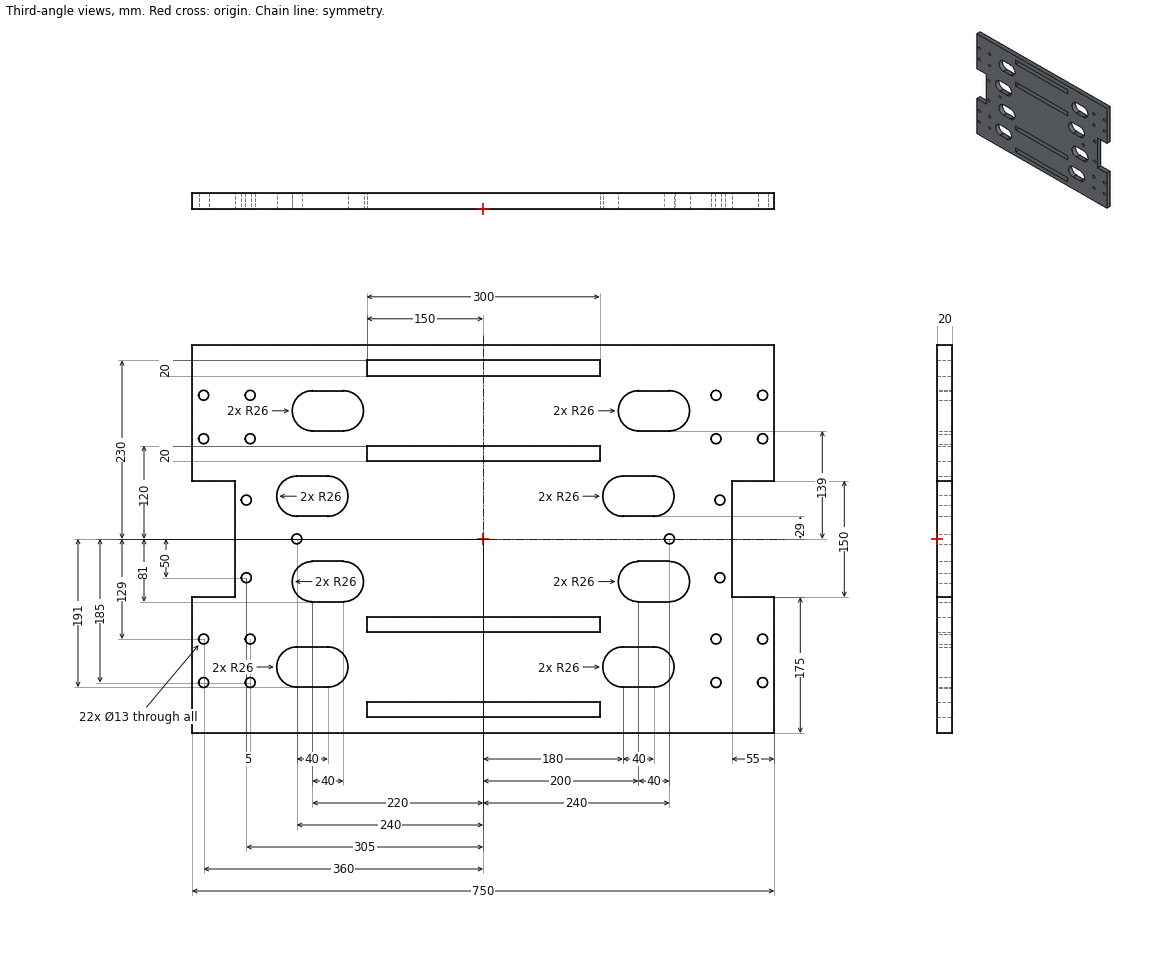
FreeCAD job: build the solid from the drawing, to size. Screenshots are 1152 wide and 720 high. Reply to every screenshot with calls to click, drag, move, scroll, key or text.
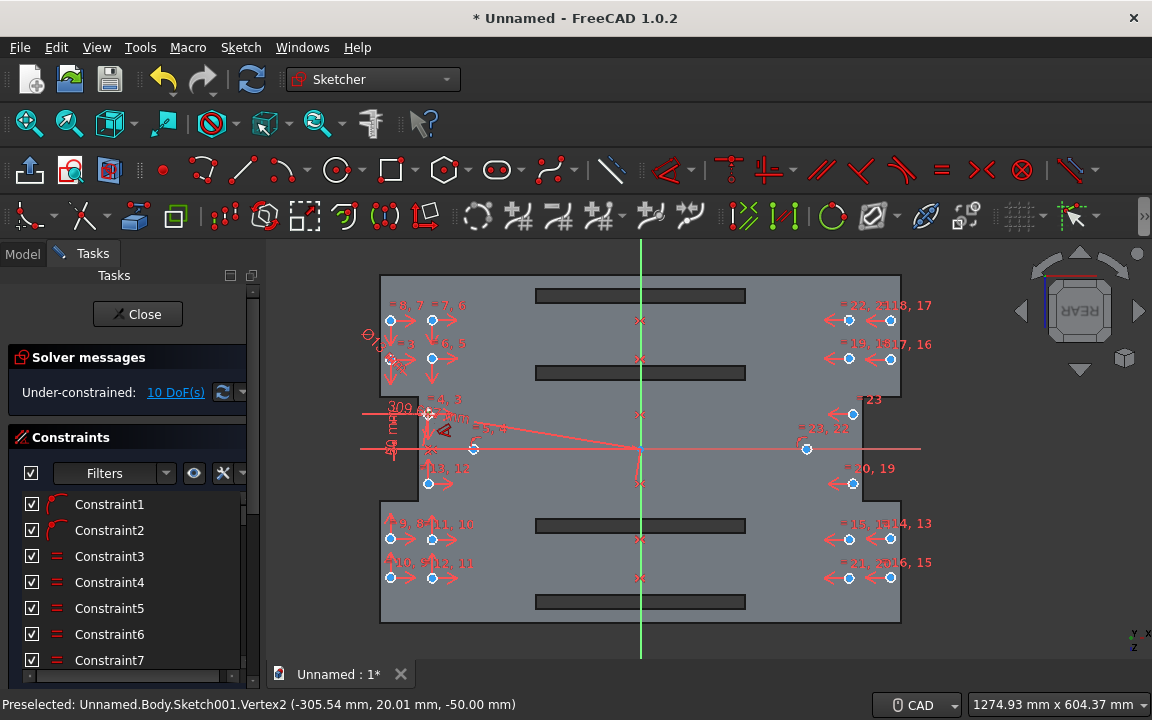
scroll(432, 359, up, 13)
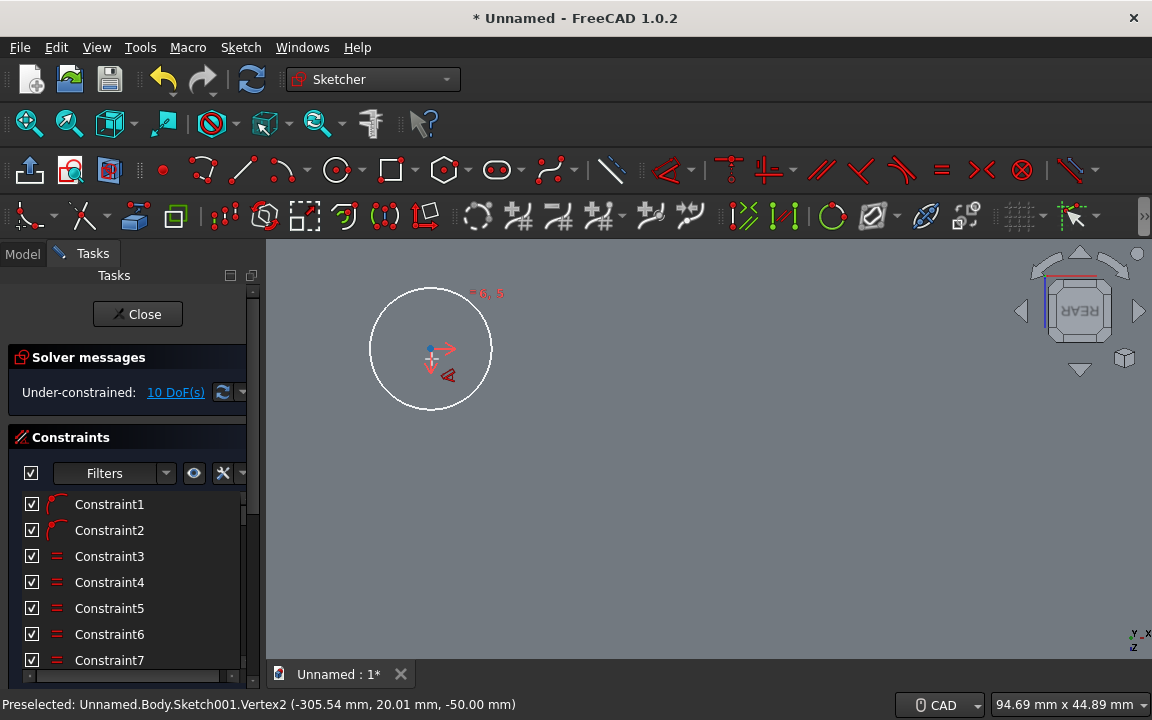
click(431, 349)
click(406, 315)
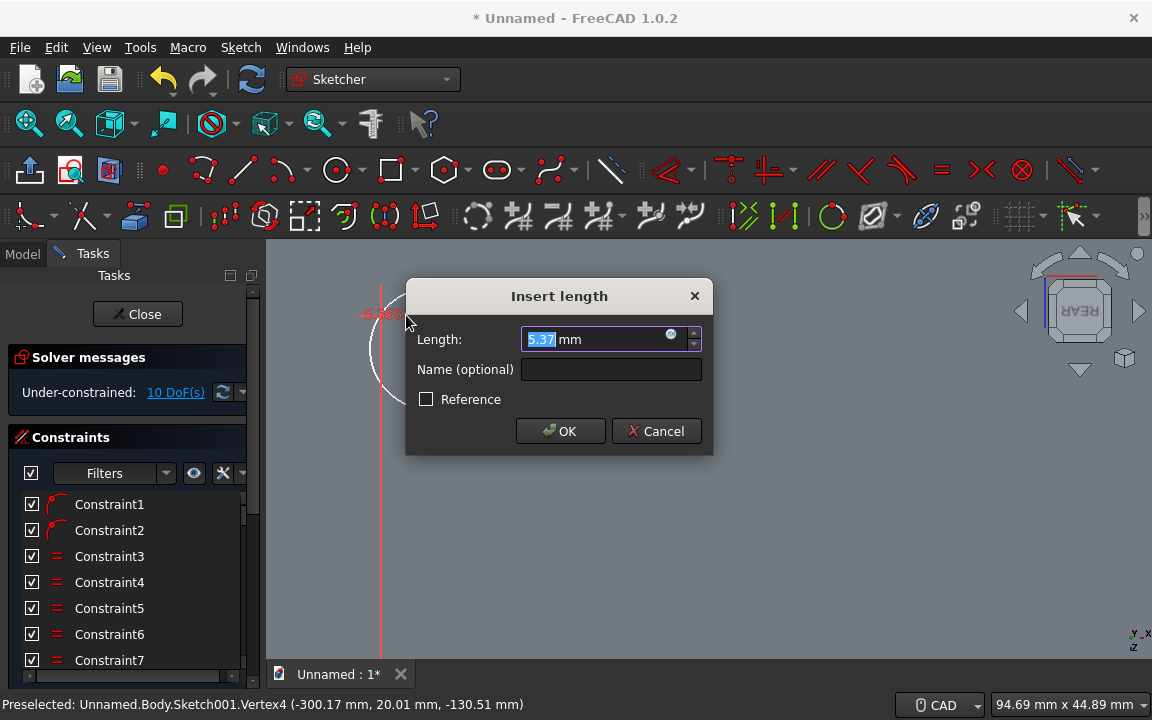
text(5)
key(Return)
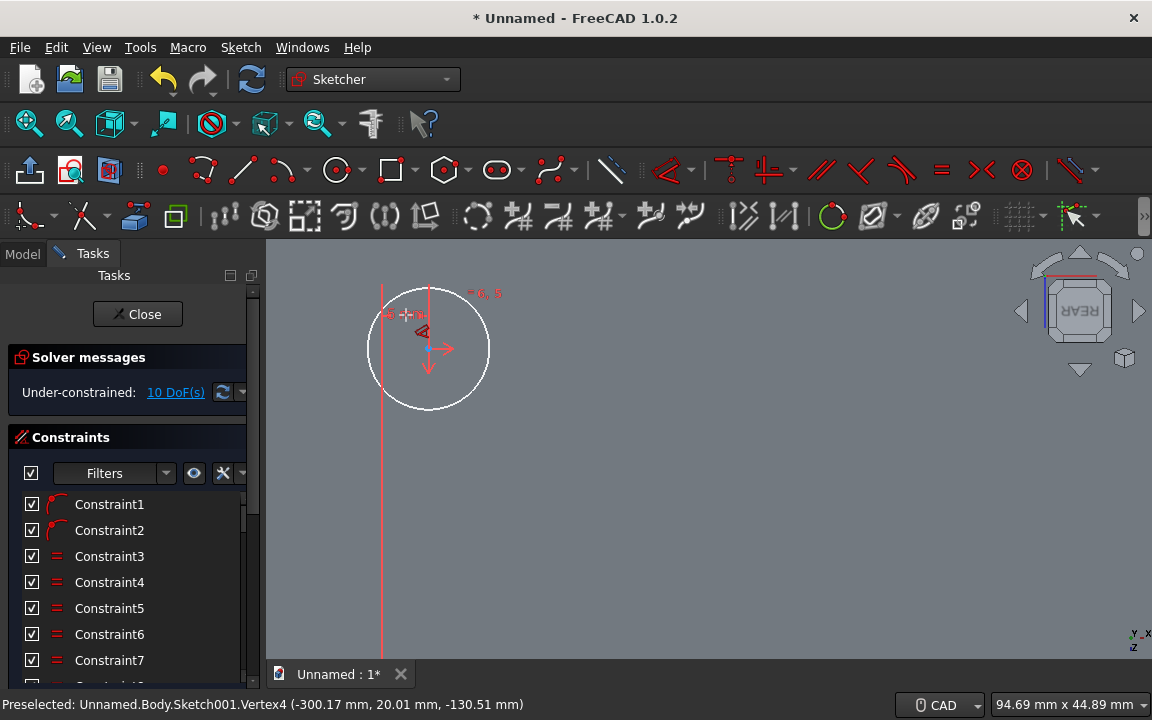
scroll(432, 359, down, 13)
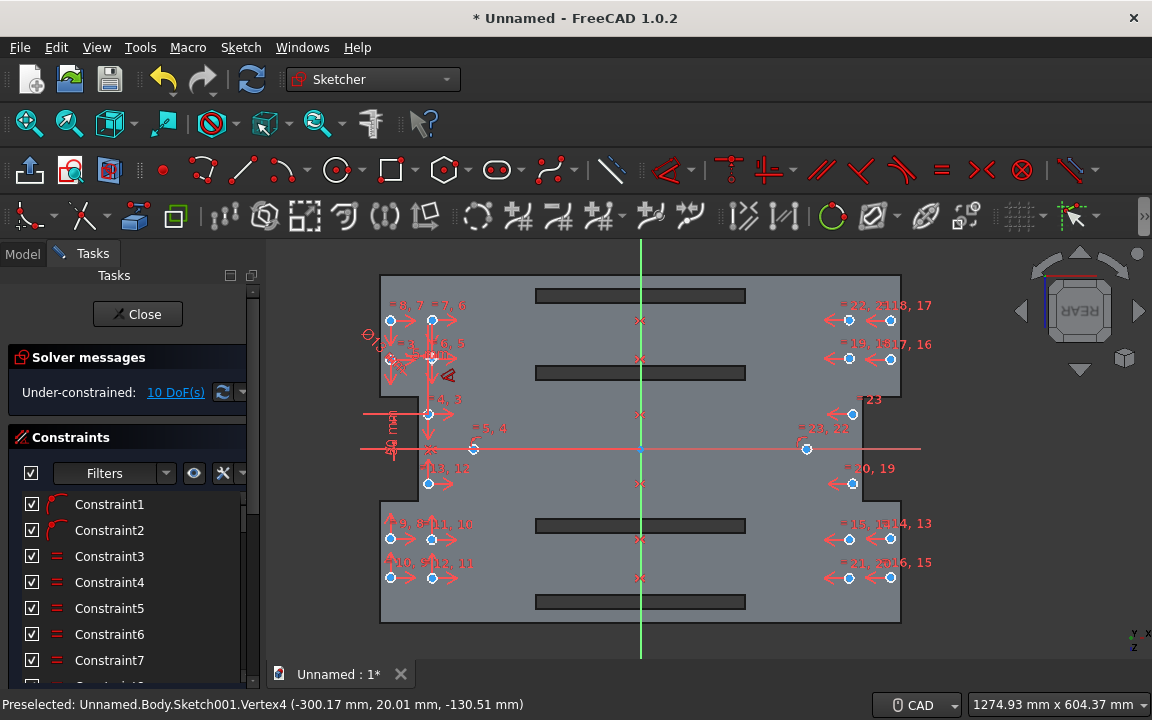
scroll(428, 414, up, 13)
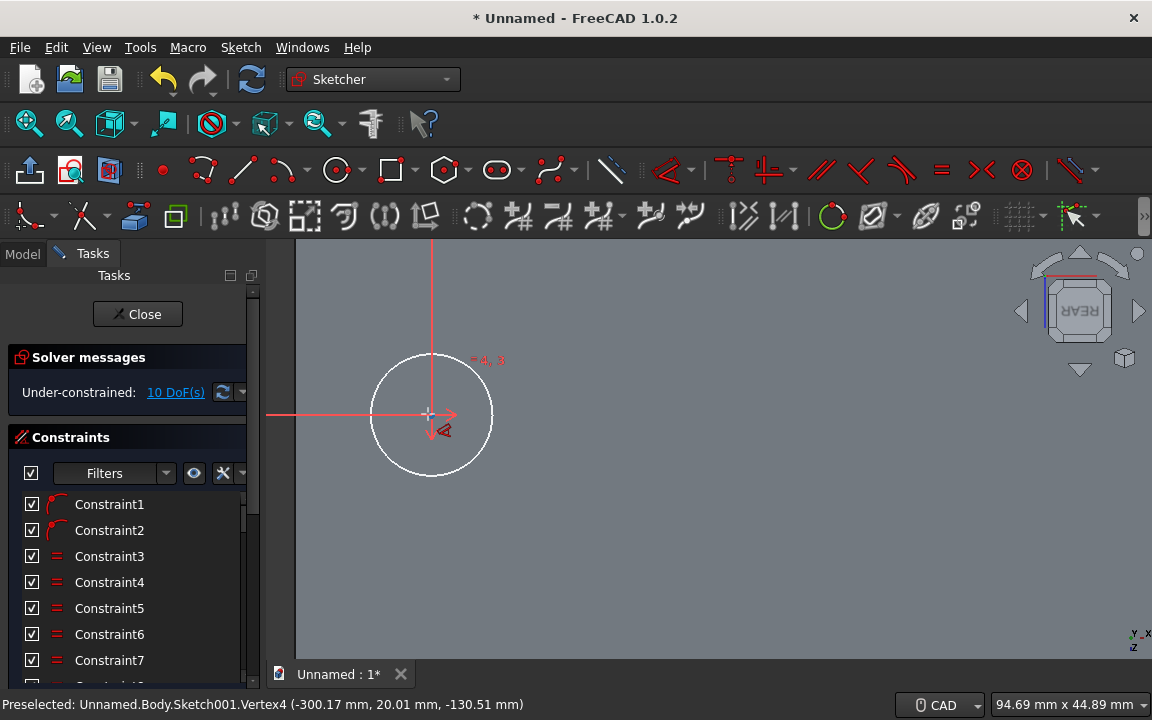
click(432, 415)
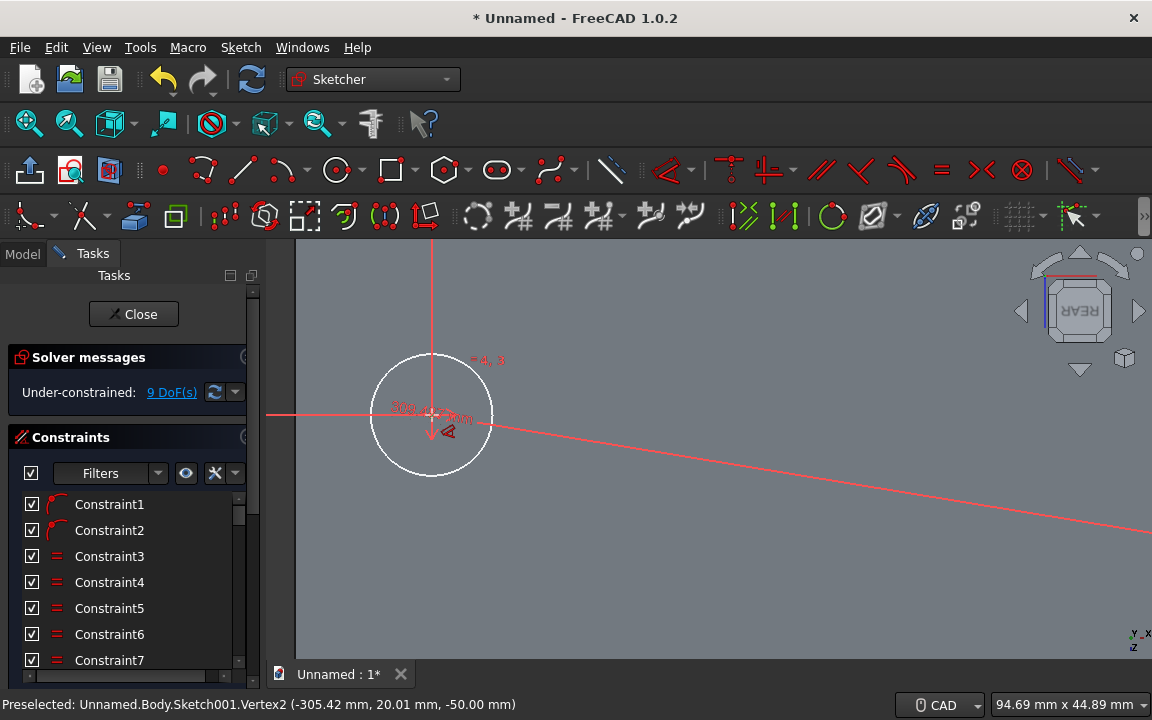
scroll(428, 414, down, 13)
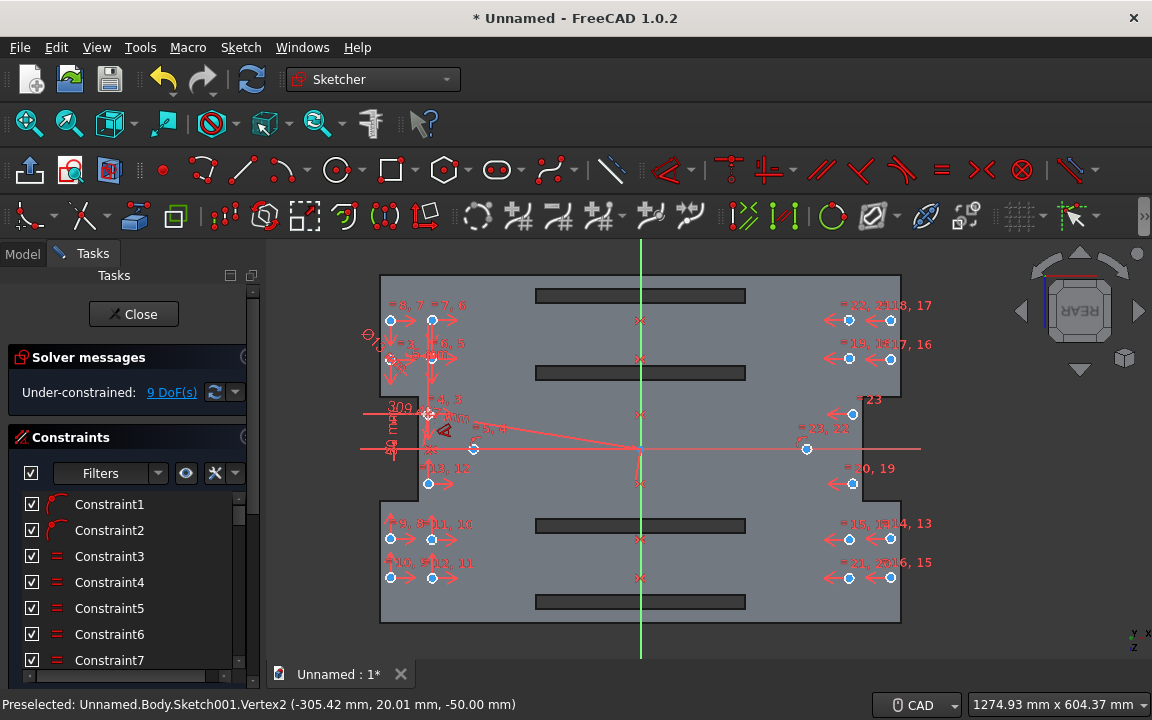
scroll(432, 320, up, 13)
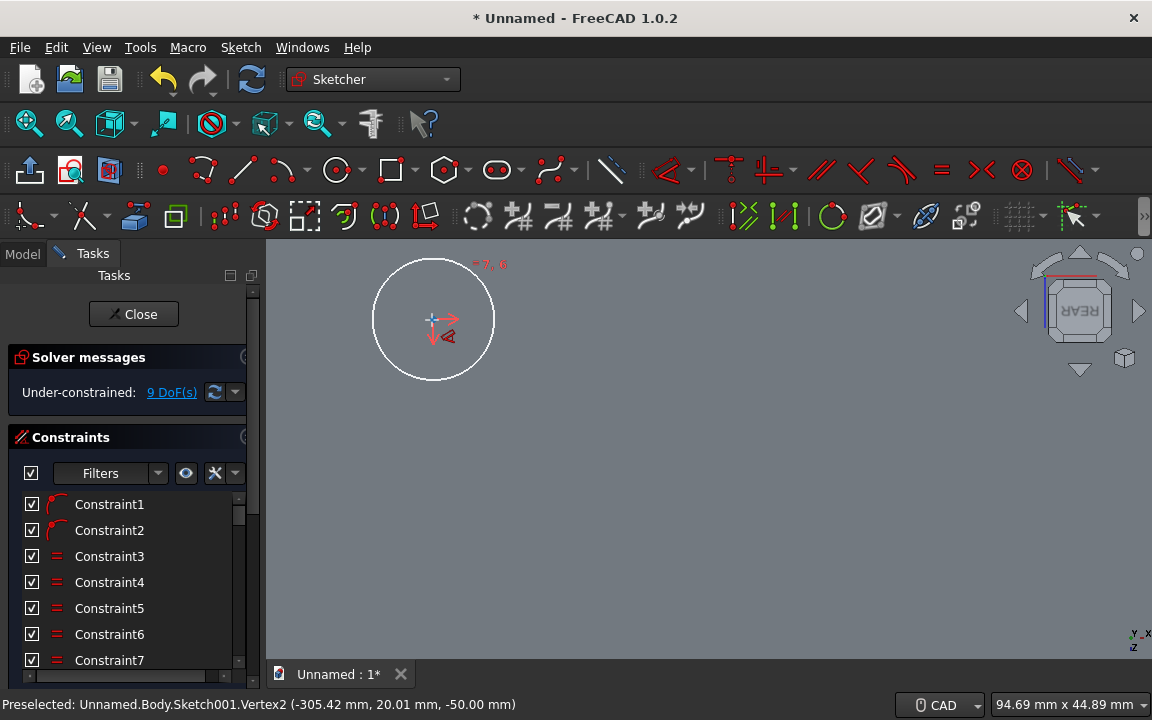
click(433, 319)
click(408, 285)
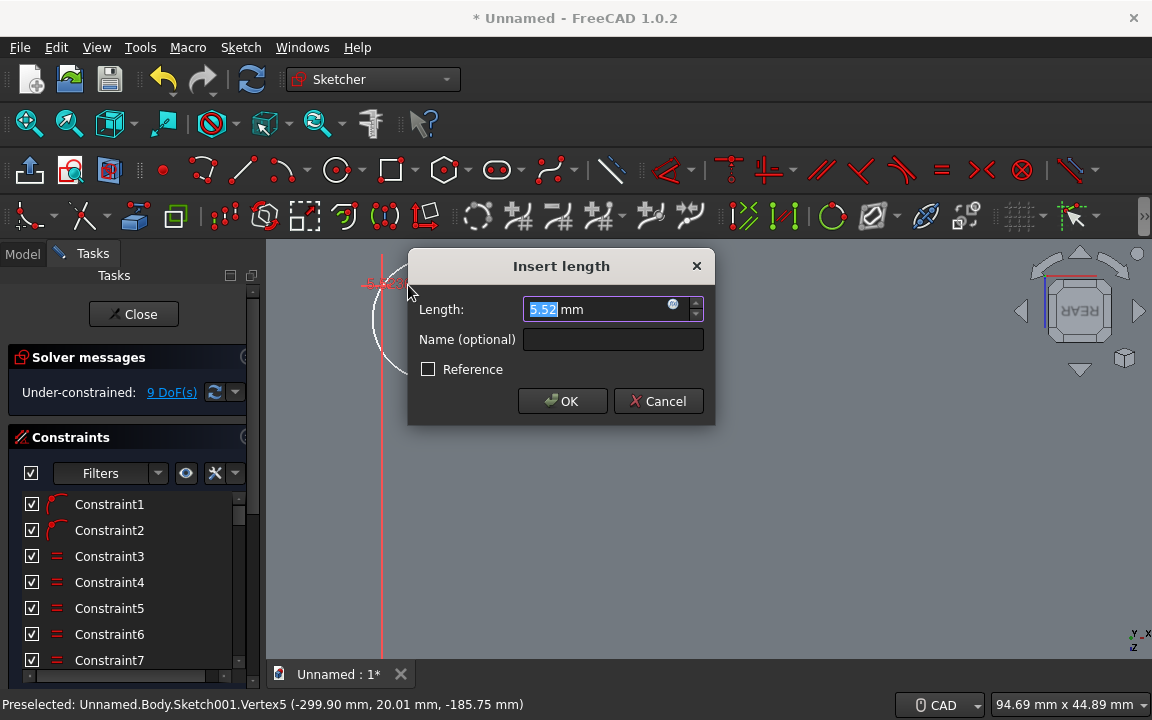
text(5)
key(Return)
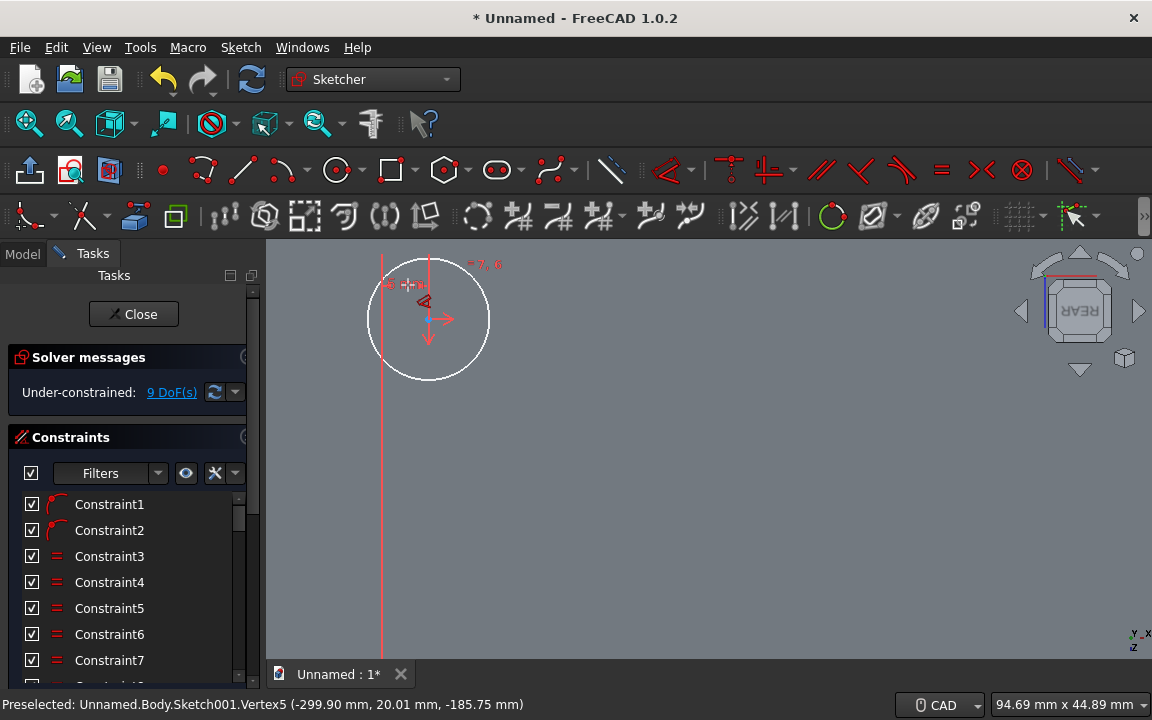
scroll(432, 320, down, 13)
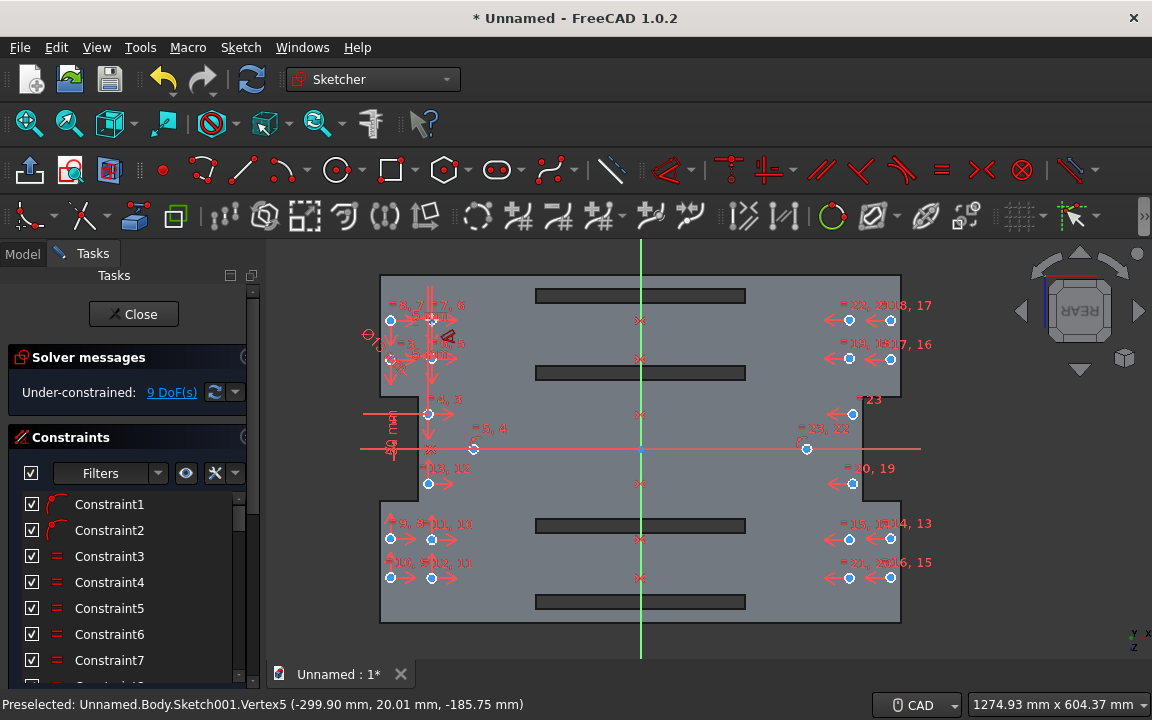
click(391, 360)
click(516, 326)